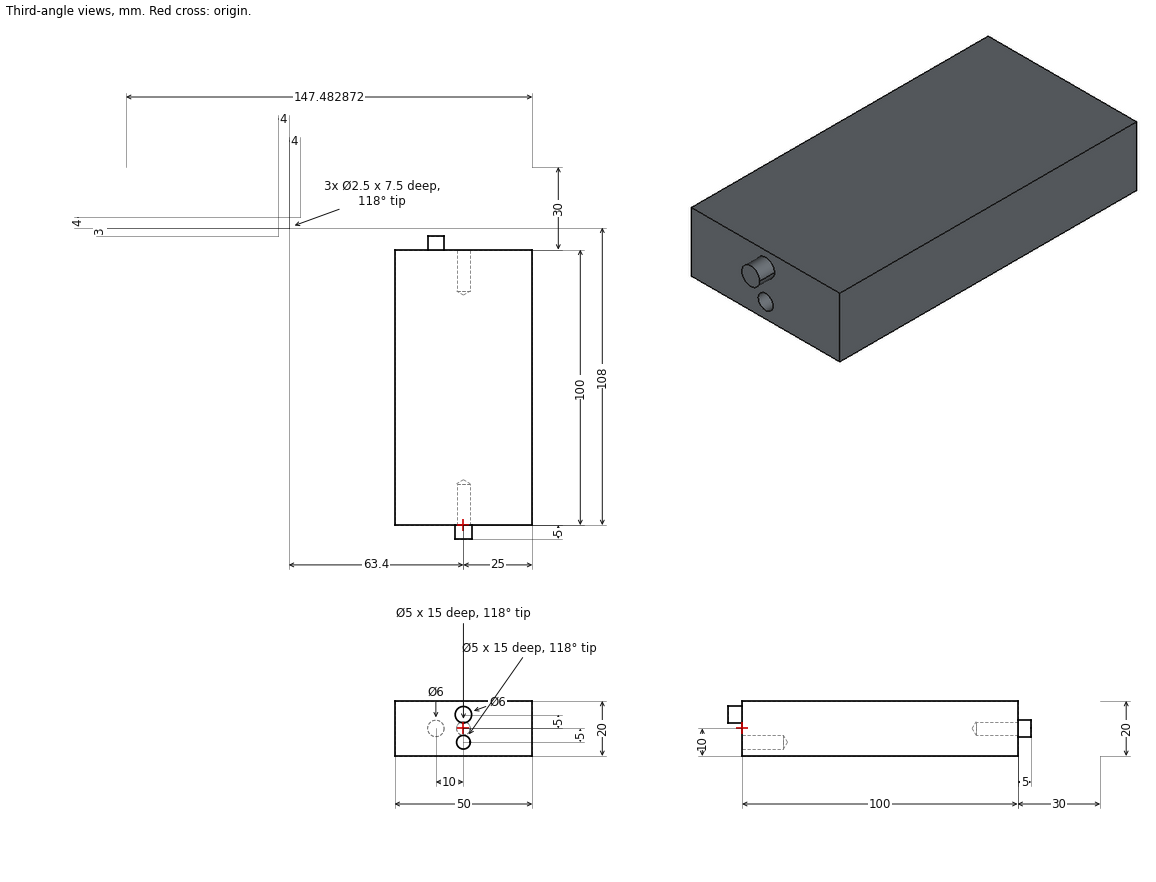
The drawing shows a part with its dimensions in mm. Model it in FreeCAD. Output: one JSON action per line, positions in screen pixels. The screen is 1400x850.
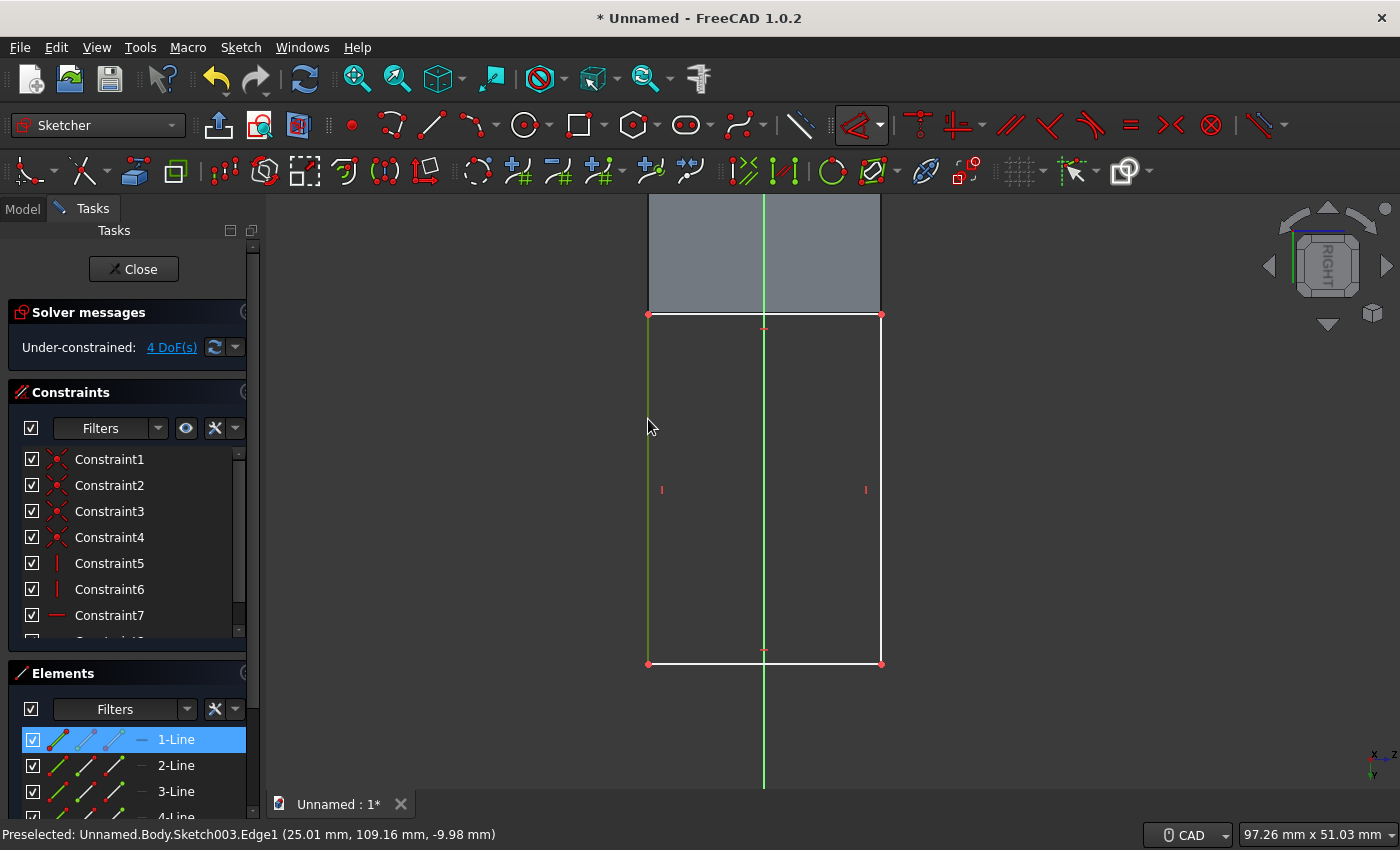
{"action": "left_click", "coordinate": [882, 126]}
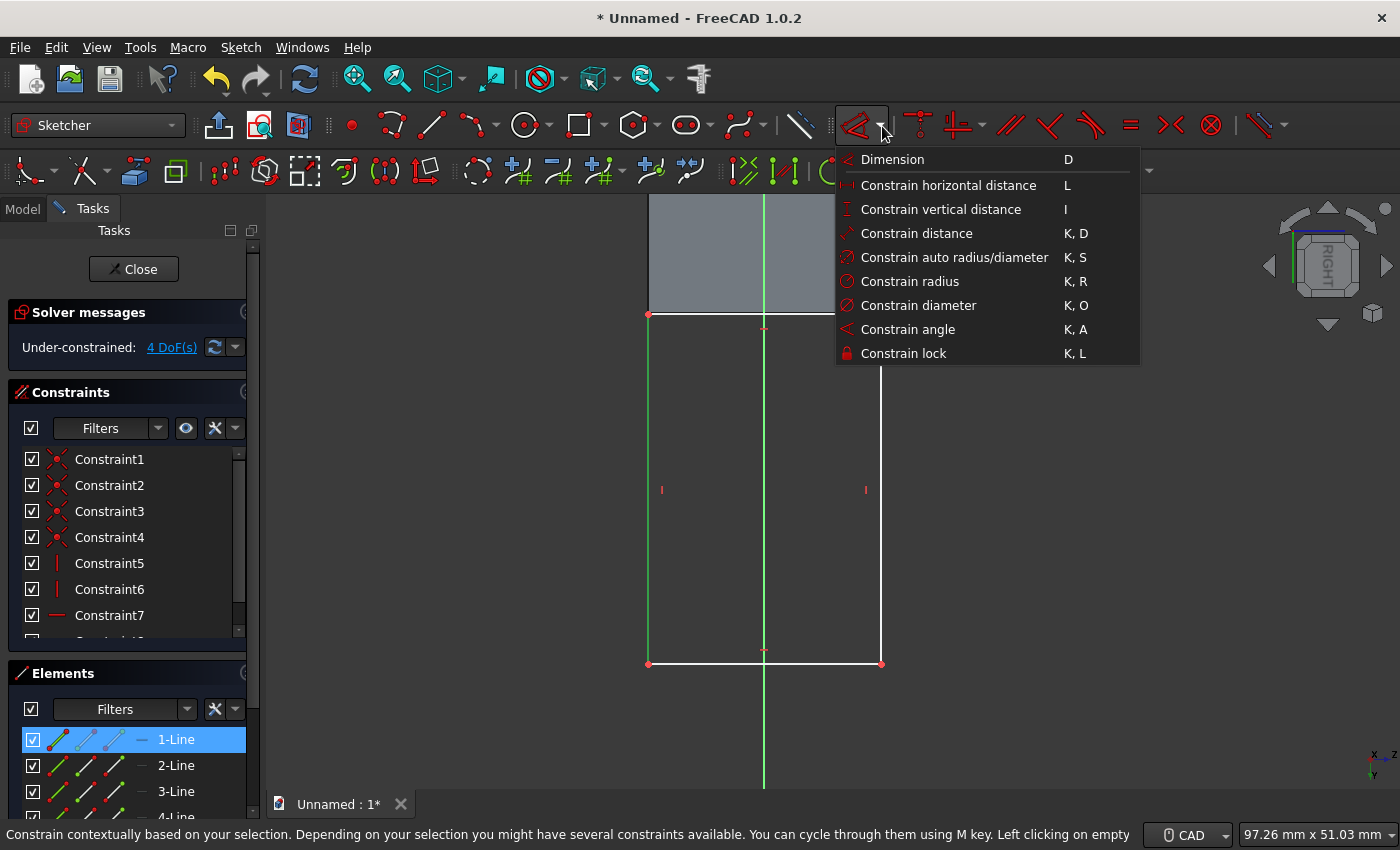
{"action": "left_click", "coordinate": [988, 209]}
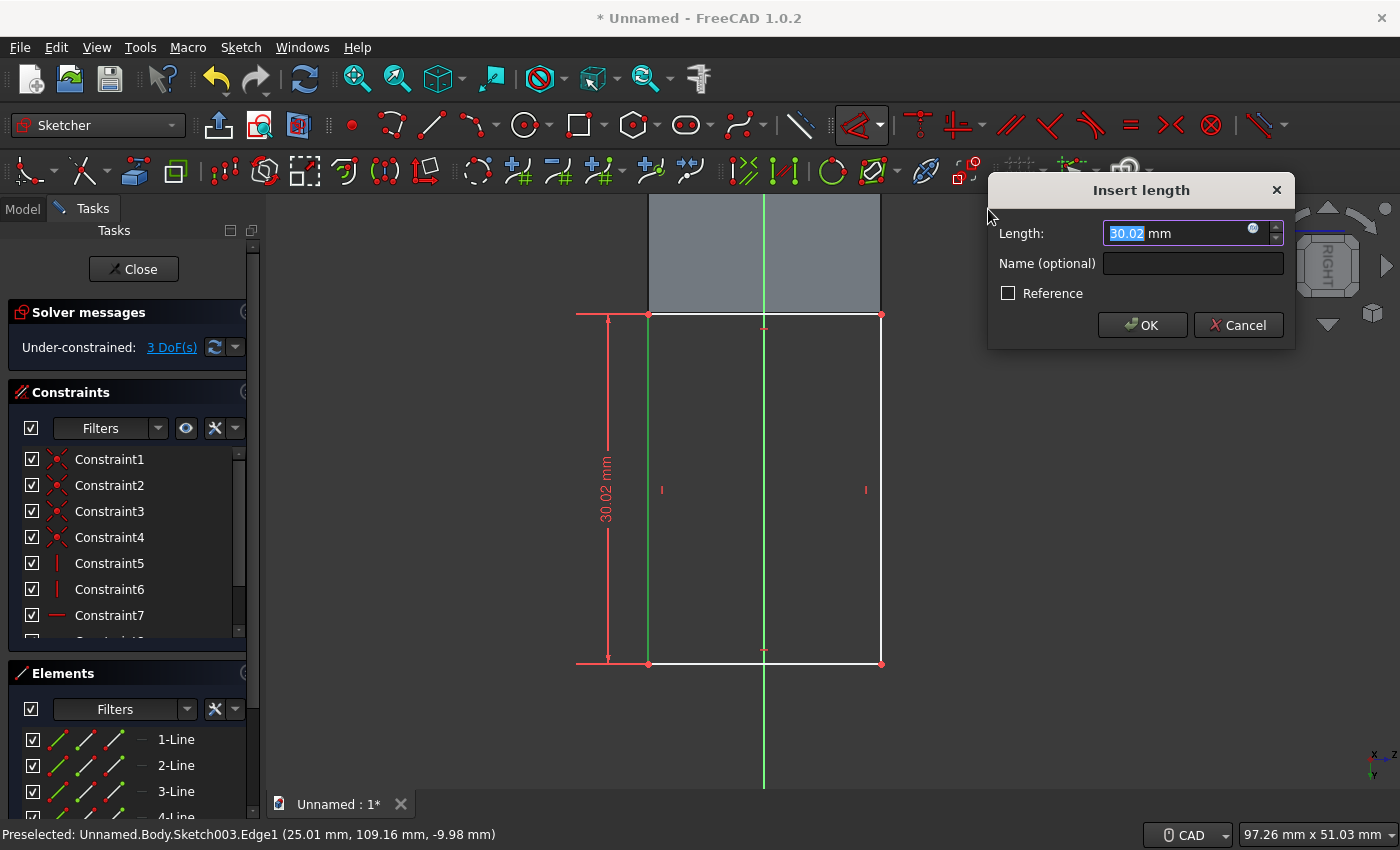
{"action": "type", "text": "30"}
{"action": "key", "text": "Return"}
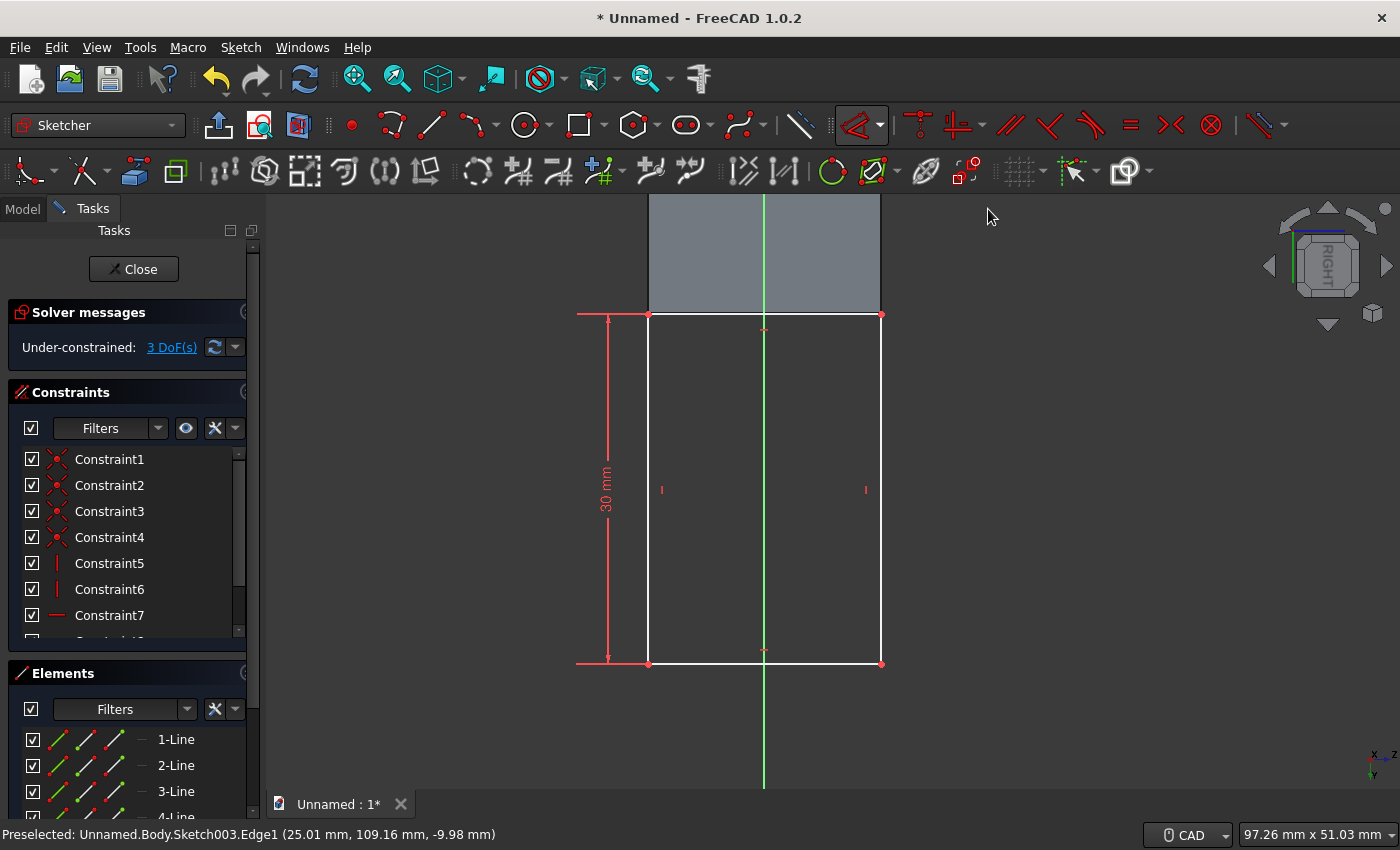
{"action": "left_click", "coordinate": [718, 664]}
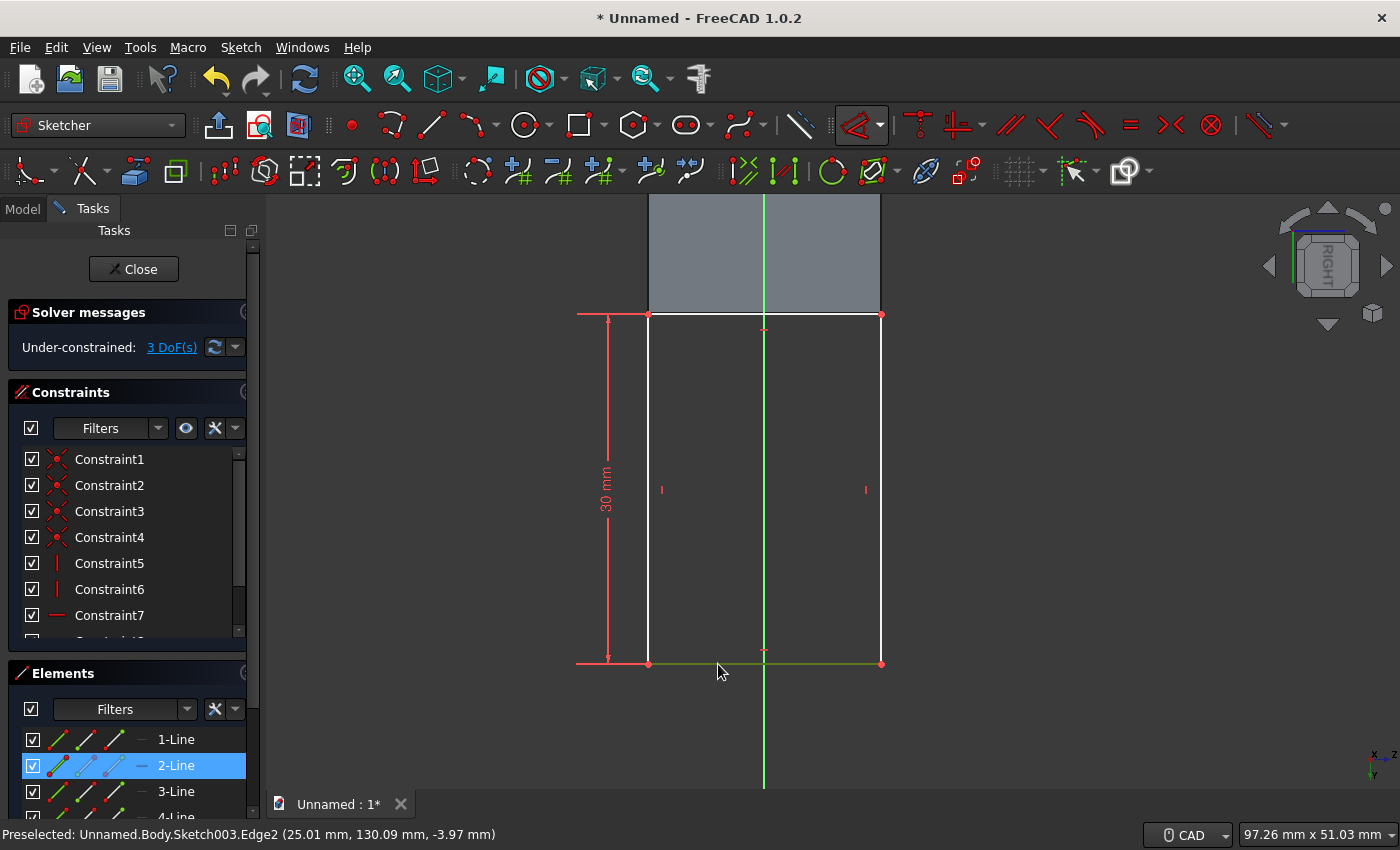
{"action": "key", "text": "l"}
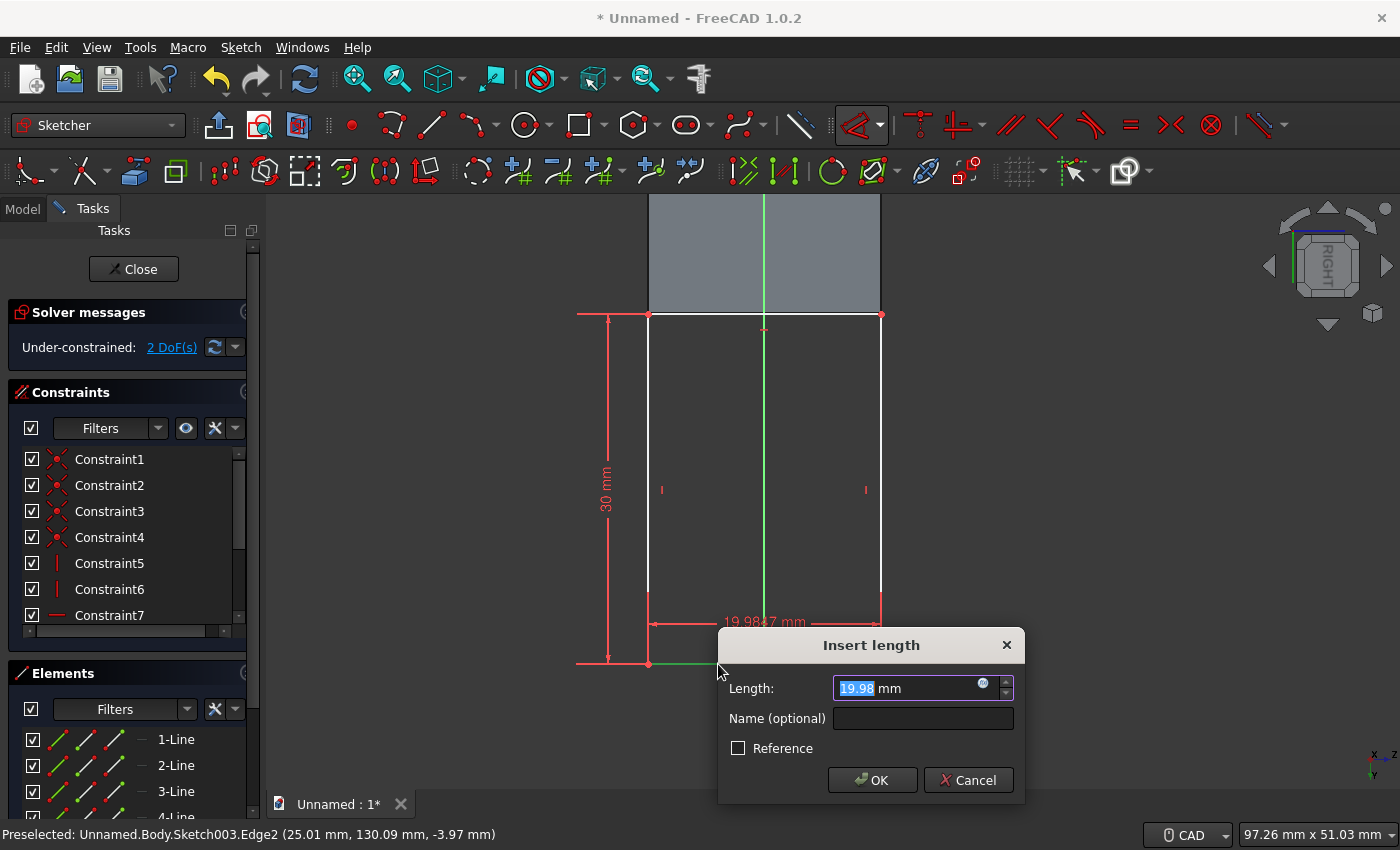
{"action": "type", "text": "20"}
{"action": "key", "text": "Return"}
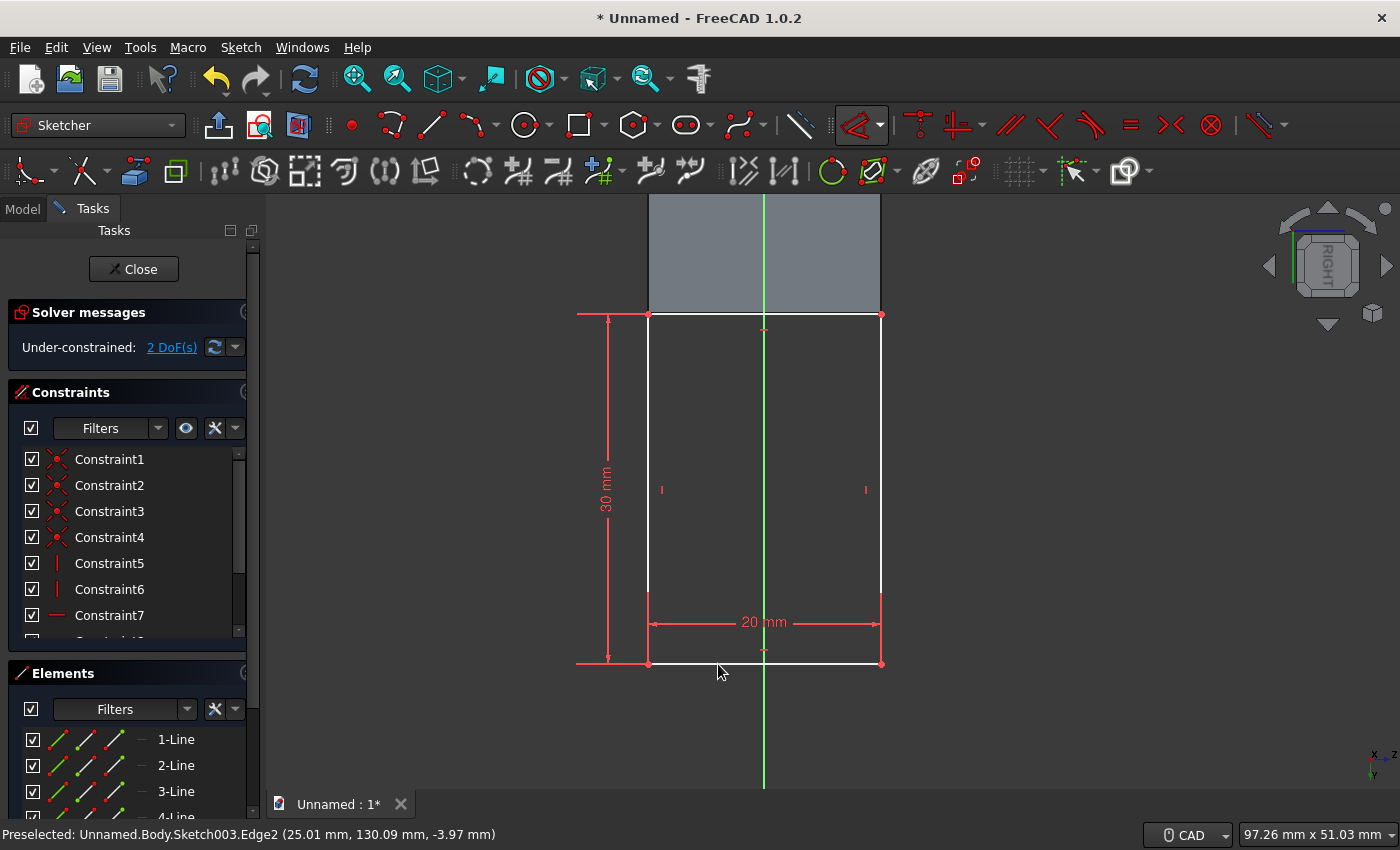
{"action": "left_click", "coordinate": [648, 314]}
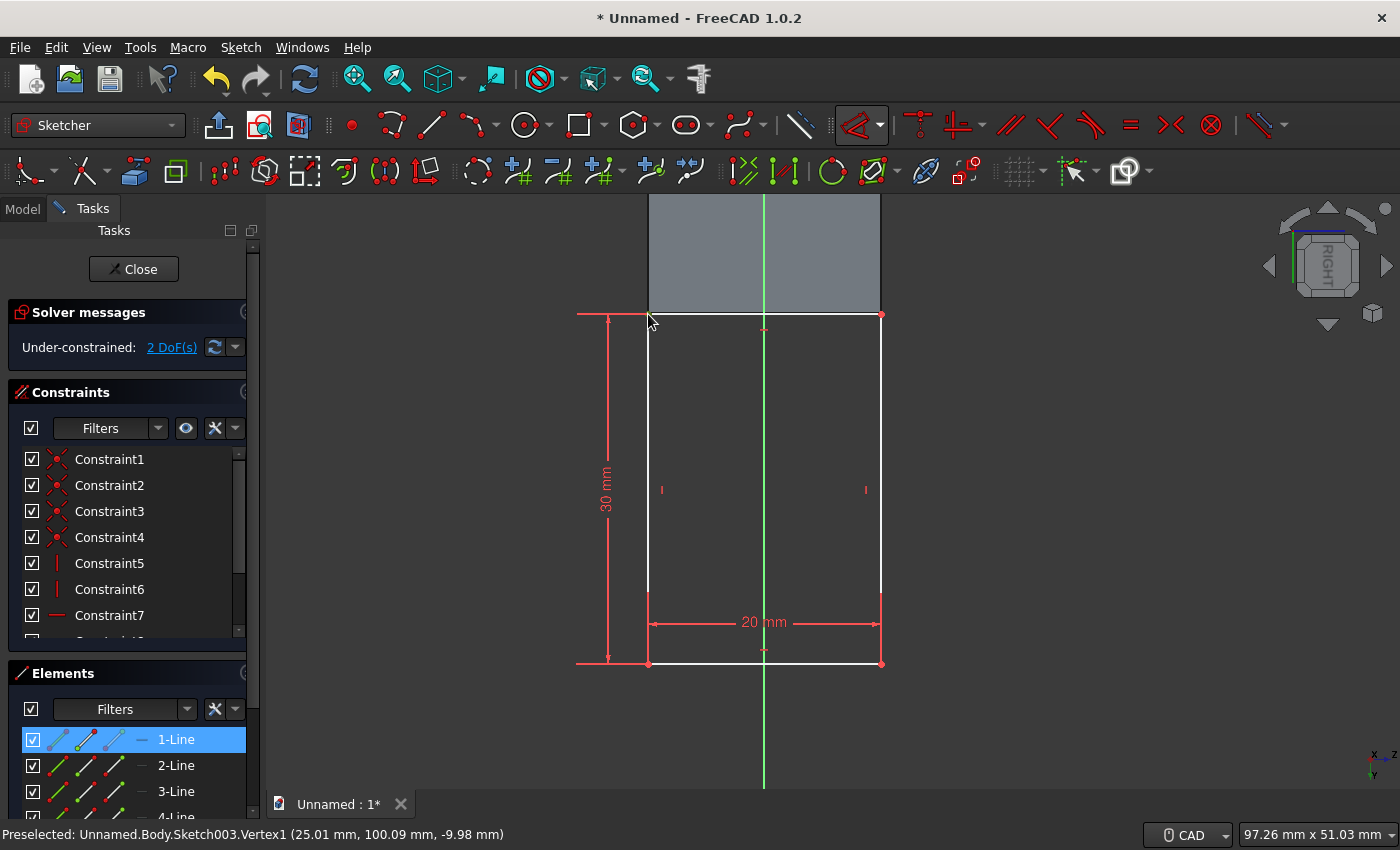
{"action": "key", "text": "l"}